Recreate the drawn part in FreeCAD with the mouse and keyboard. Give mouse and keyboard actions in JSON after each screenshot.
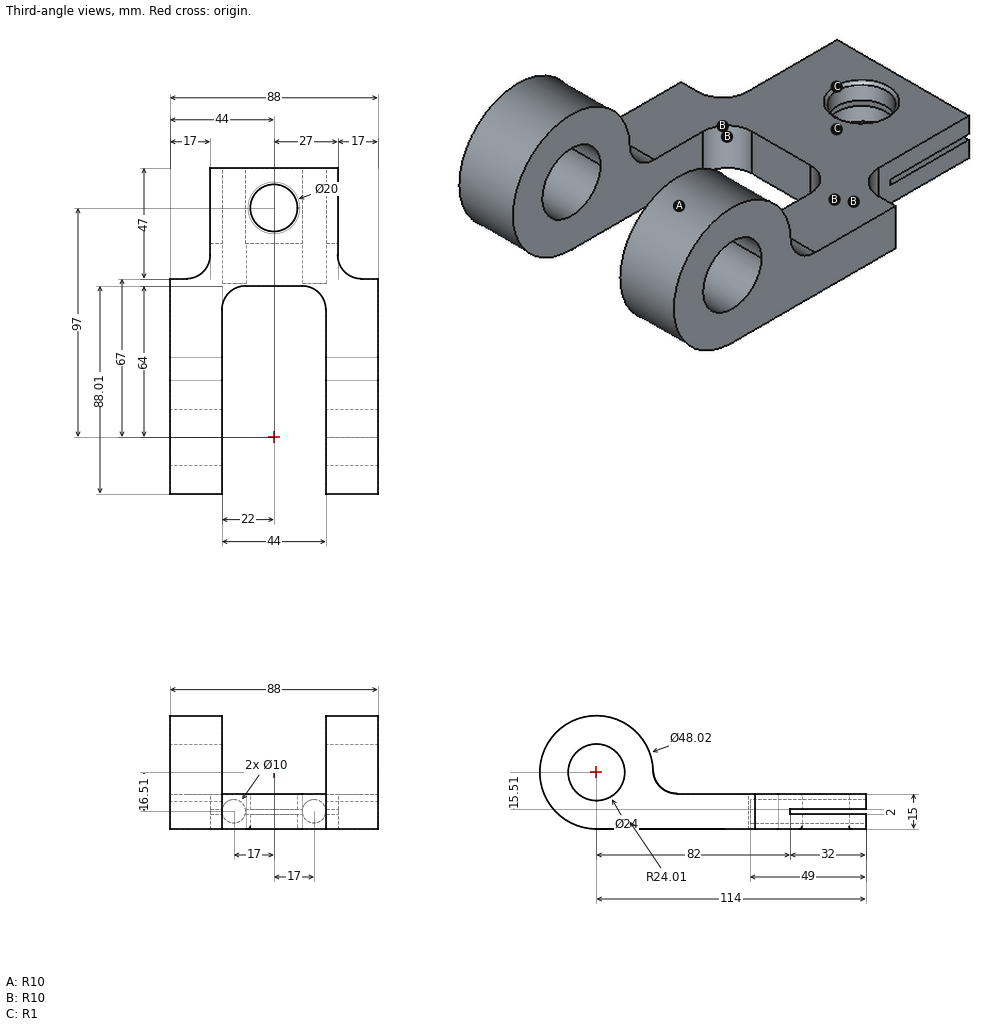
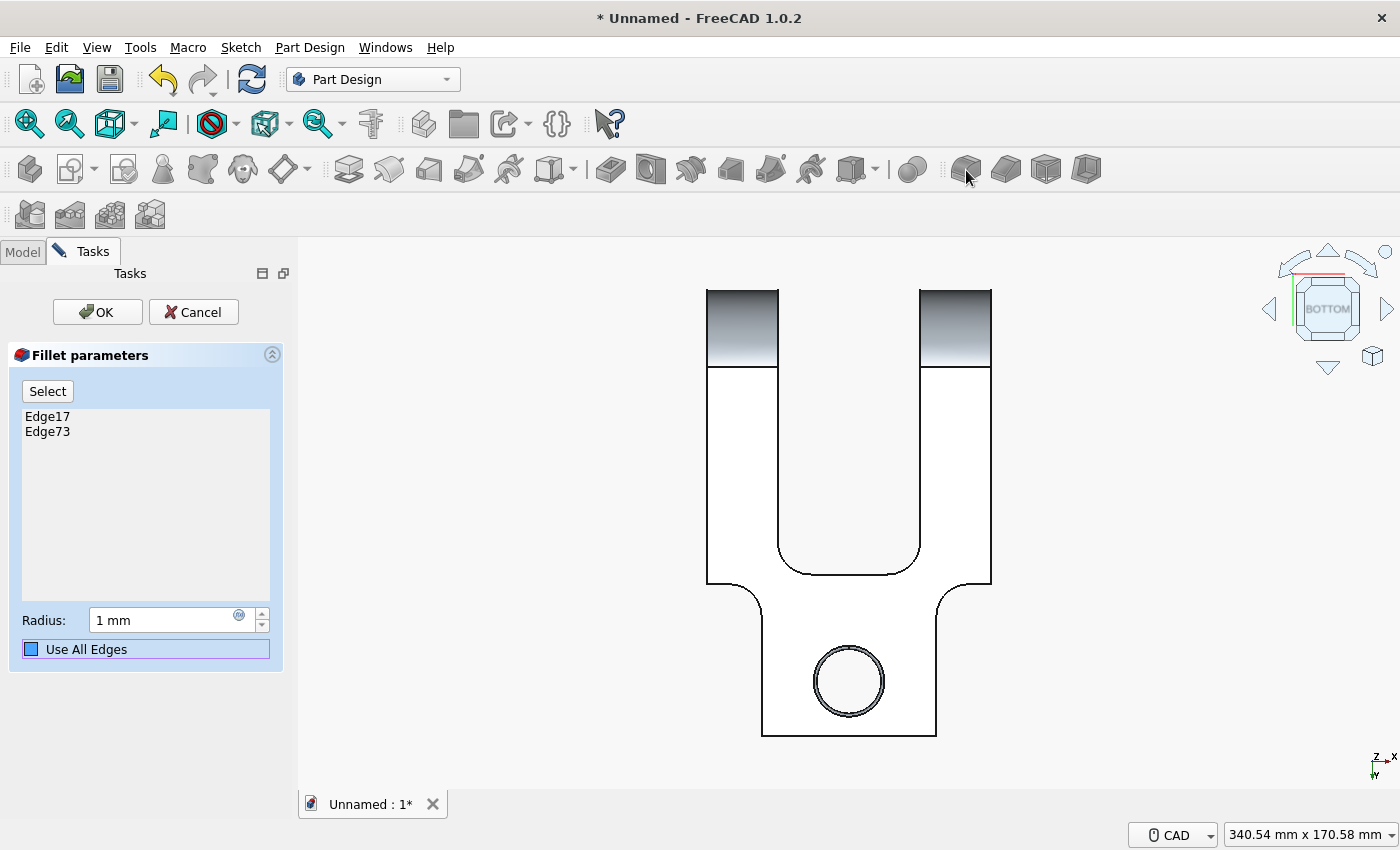
{"action": "left_click", "coordinate": [98, 312]}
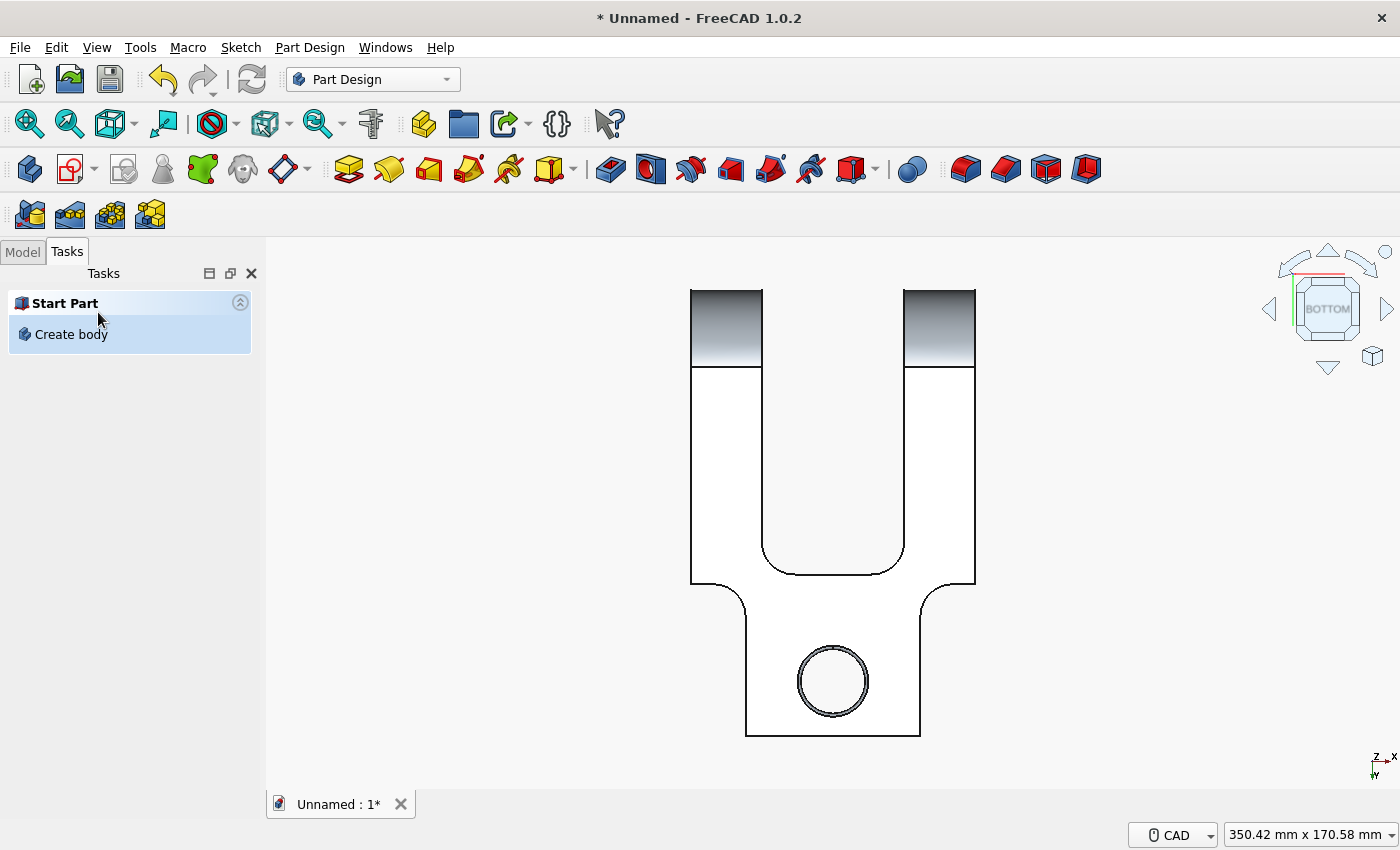
{"action": "key", "text": "4"}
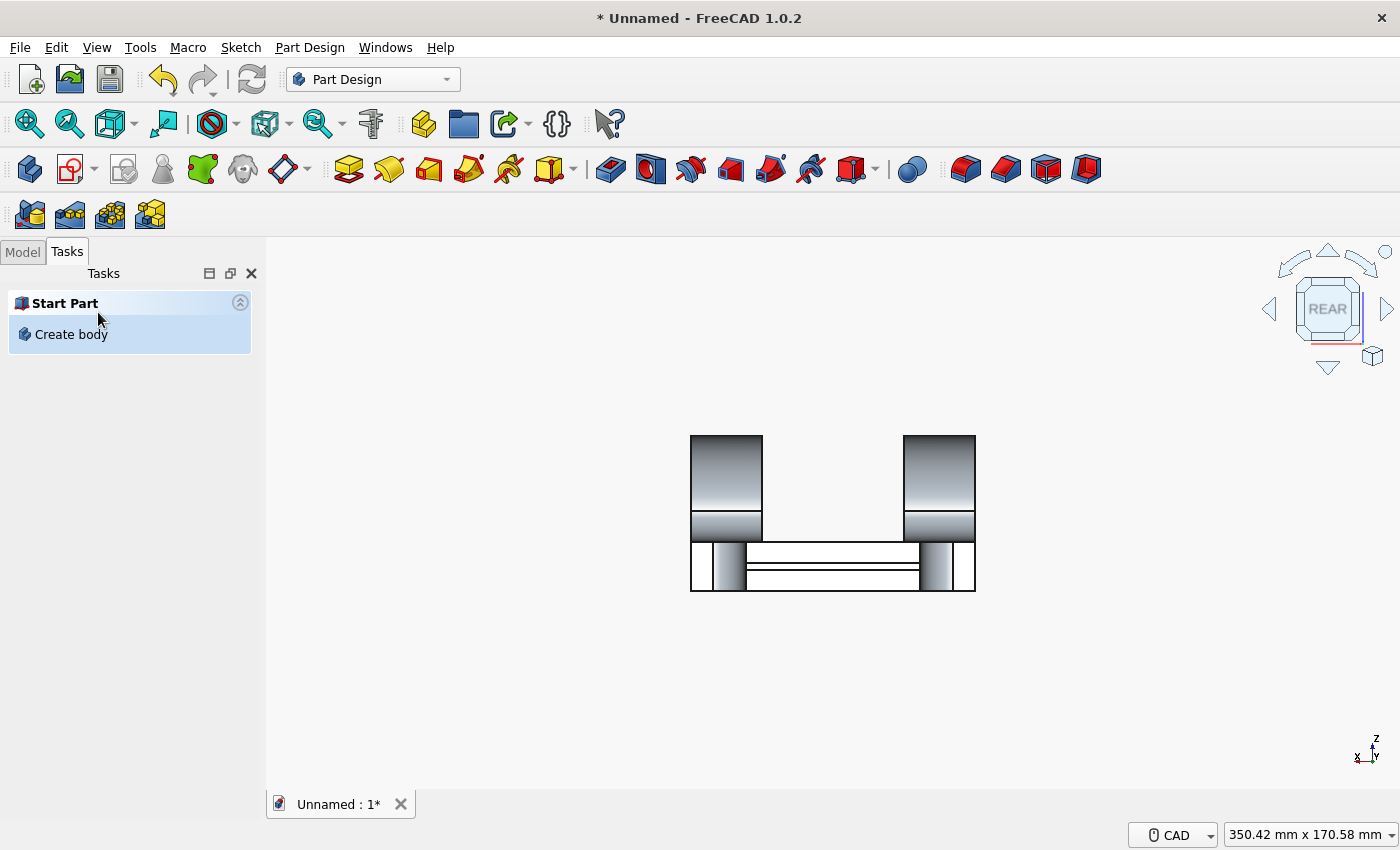
{"action": "left_click", "coordinate": [30, 124]}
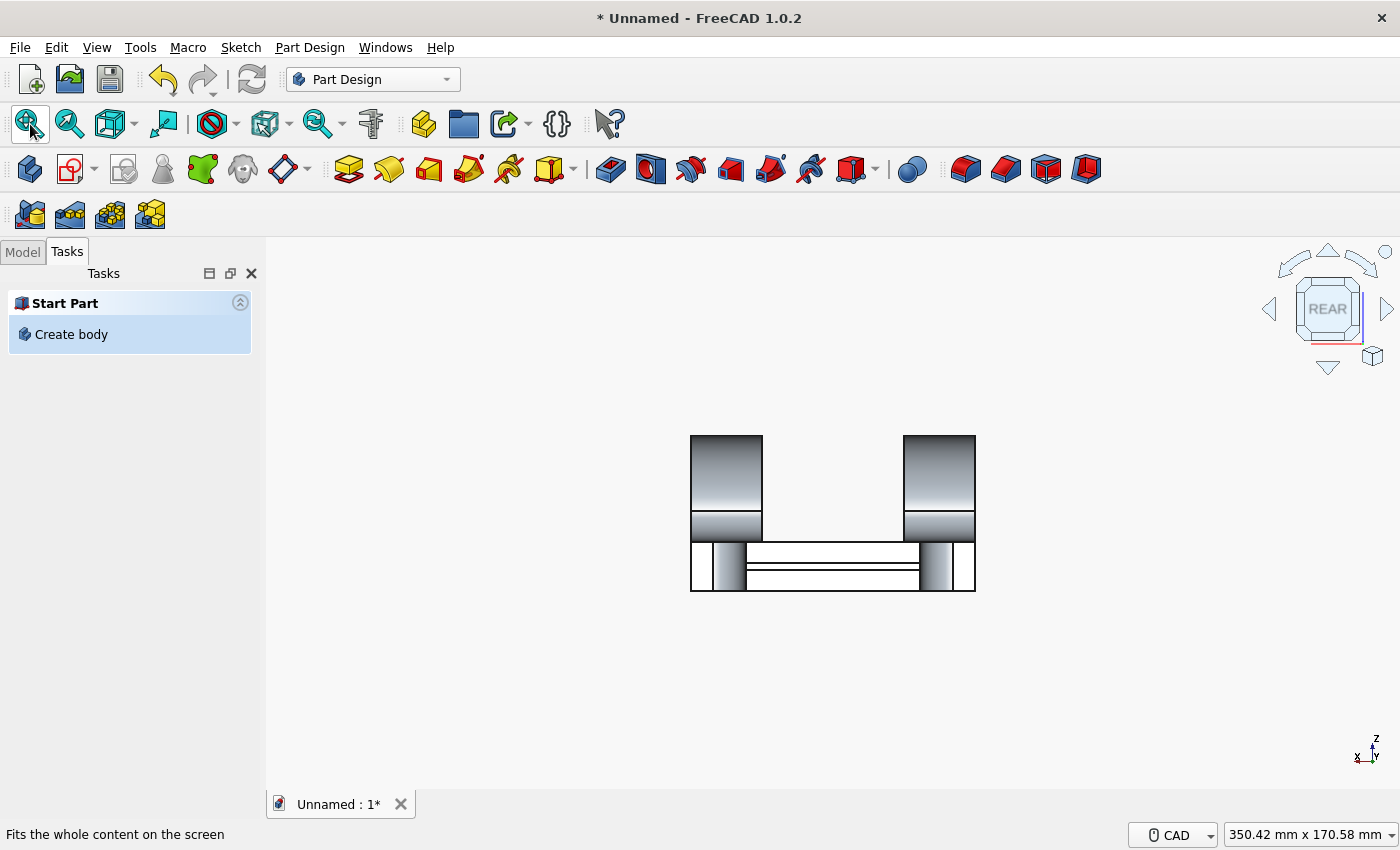
{"action": "left_click", "coordinate": [883, 579]}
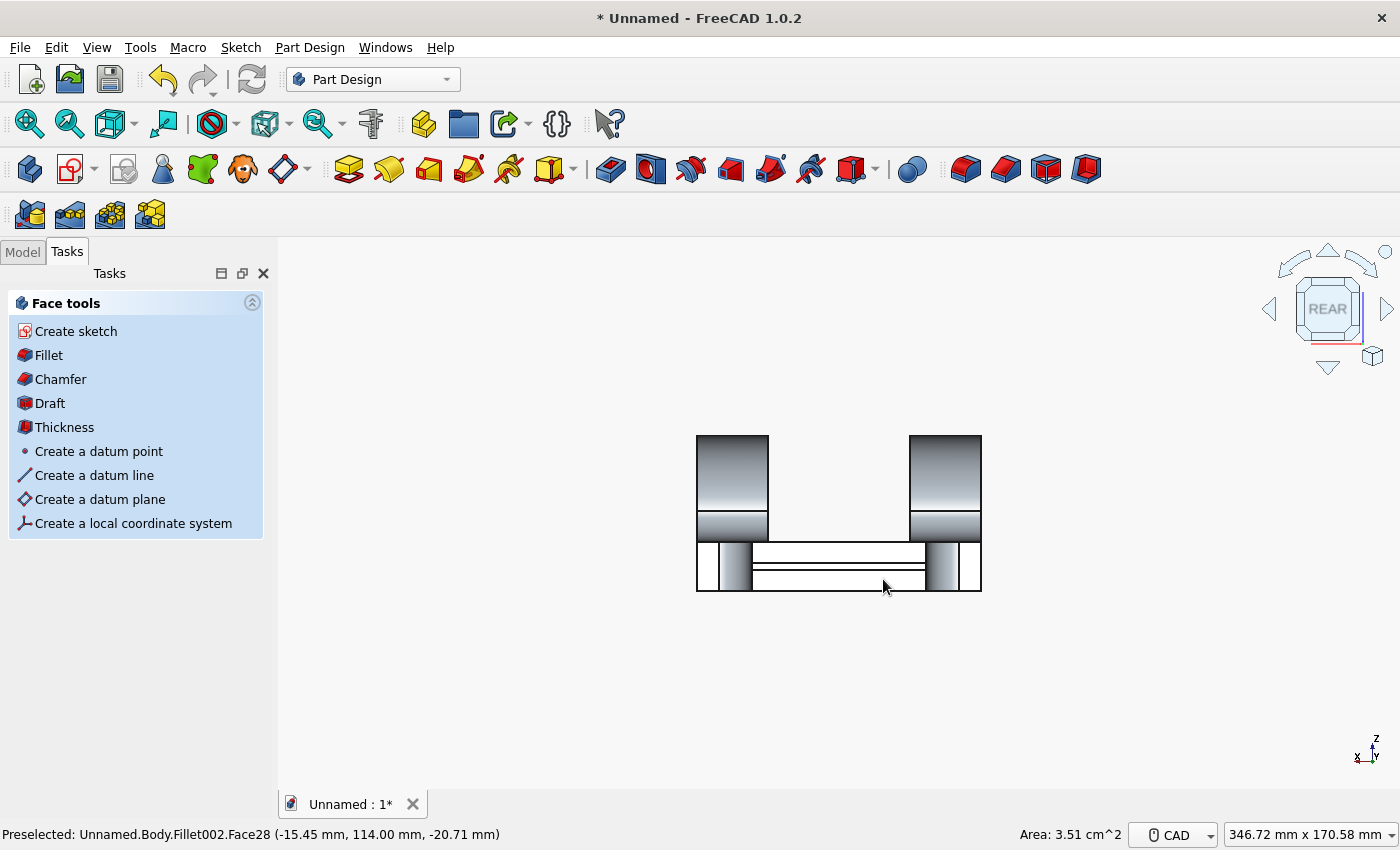
{"action": "left_click", "coordinate": [70, 170]}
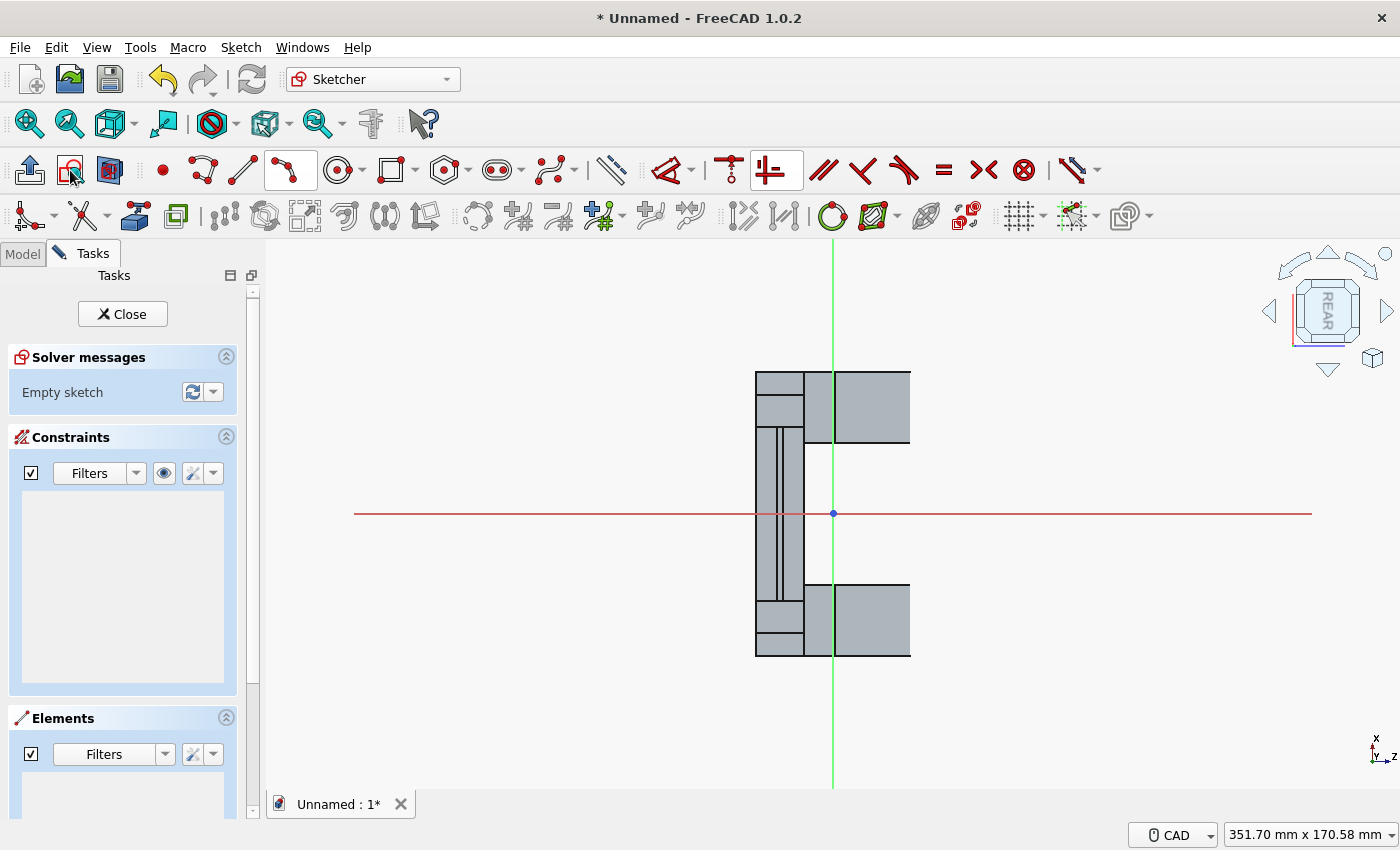
{"action": "scroll", "coordinate": [826, 514], "scroll_direction": "up", "scroll_amount": 4}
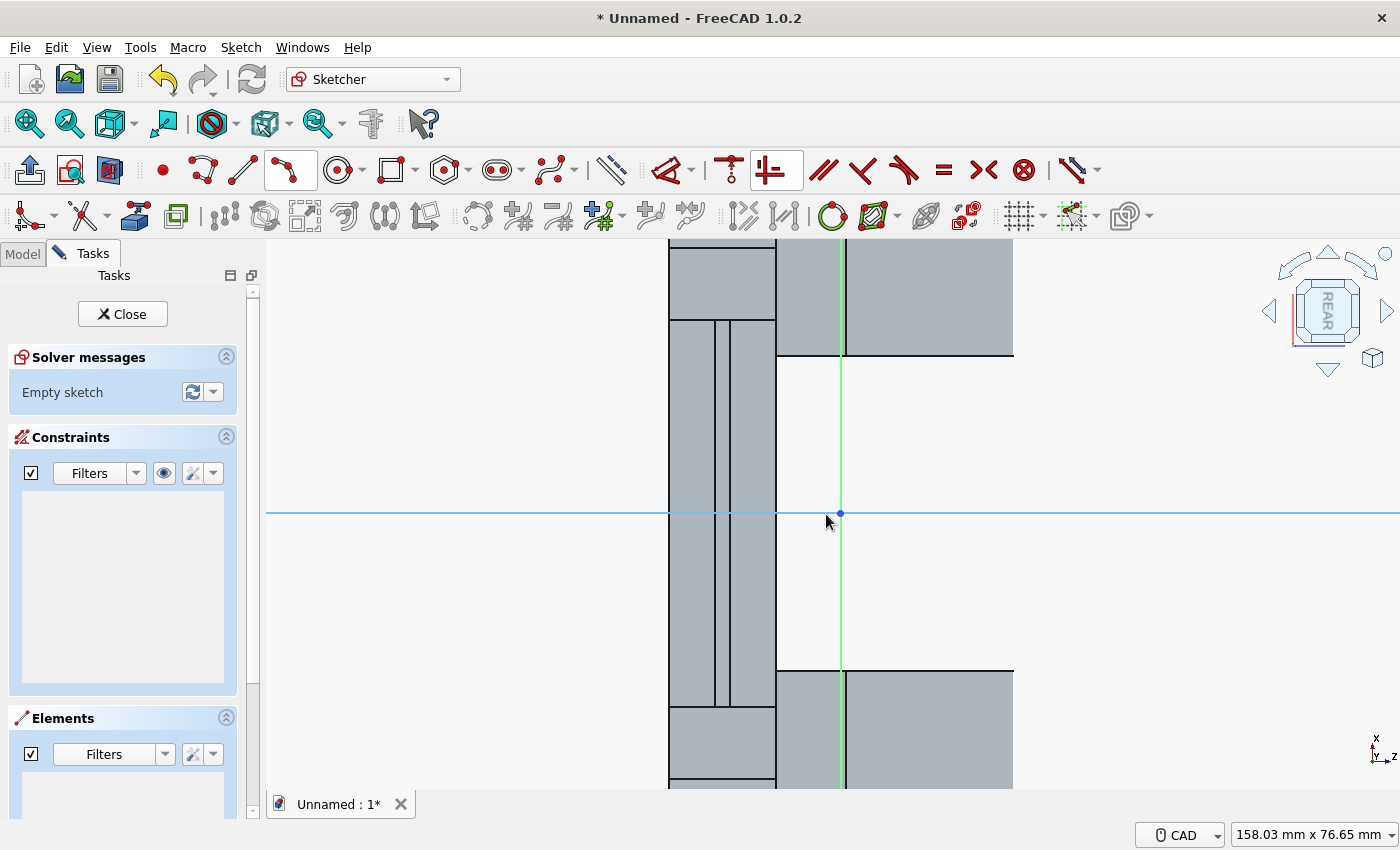
{"action": "left_click", "coordinate": [338, 170]}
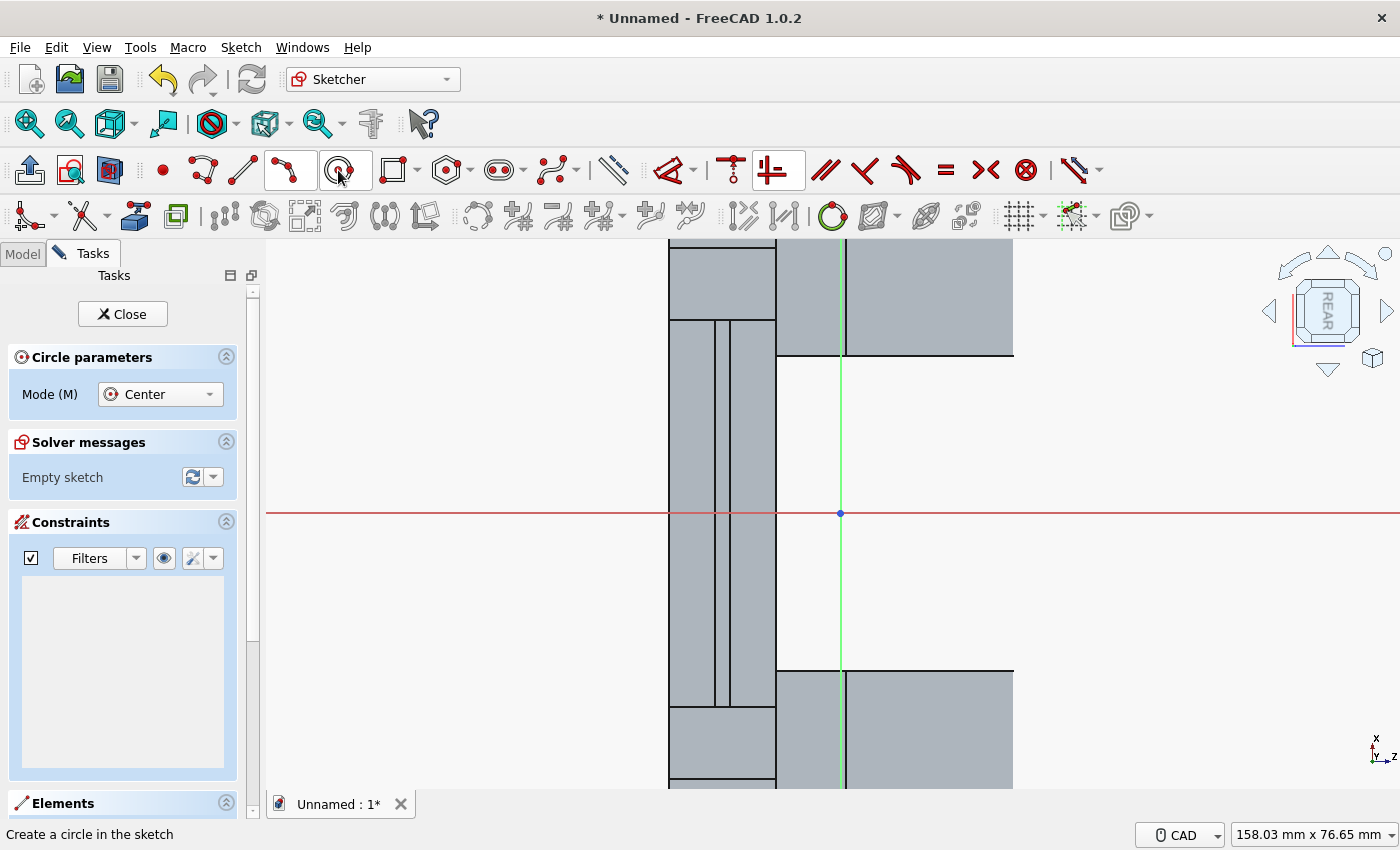
{"action": "left_click", "coordinate": [723, 635]}
{"action": "left_click", "coordinate": [748, 610]}